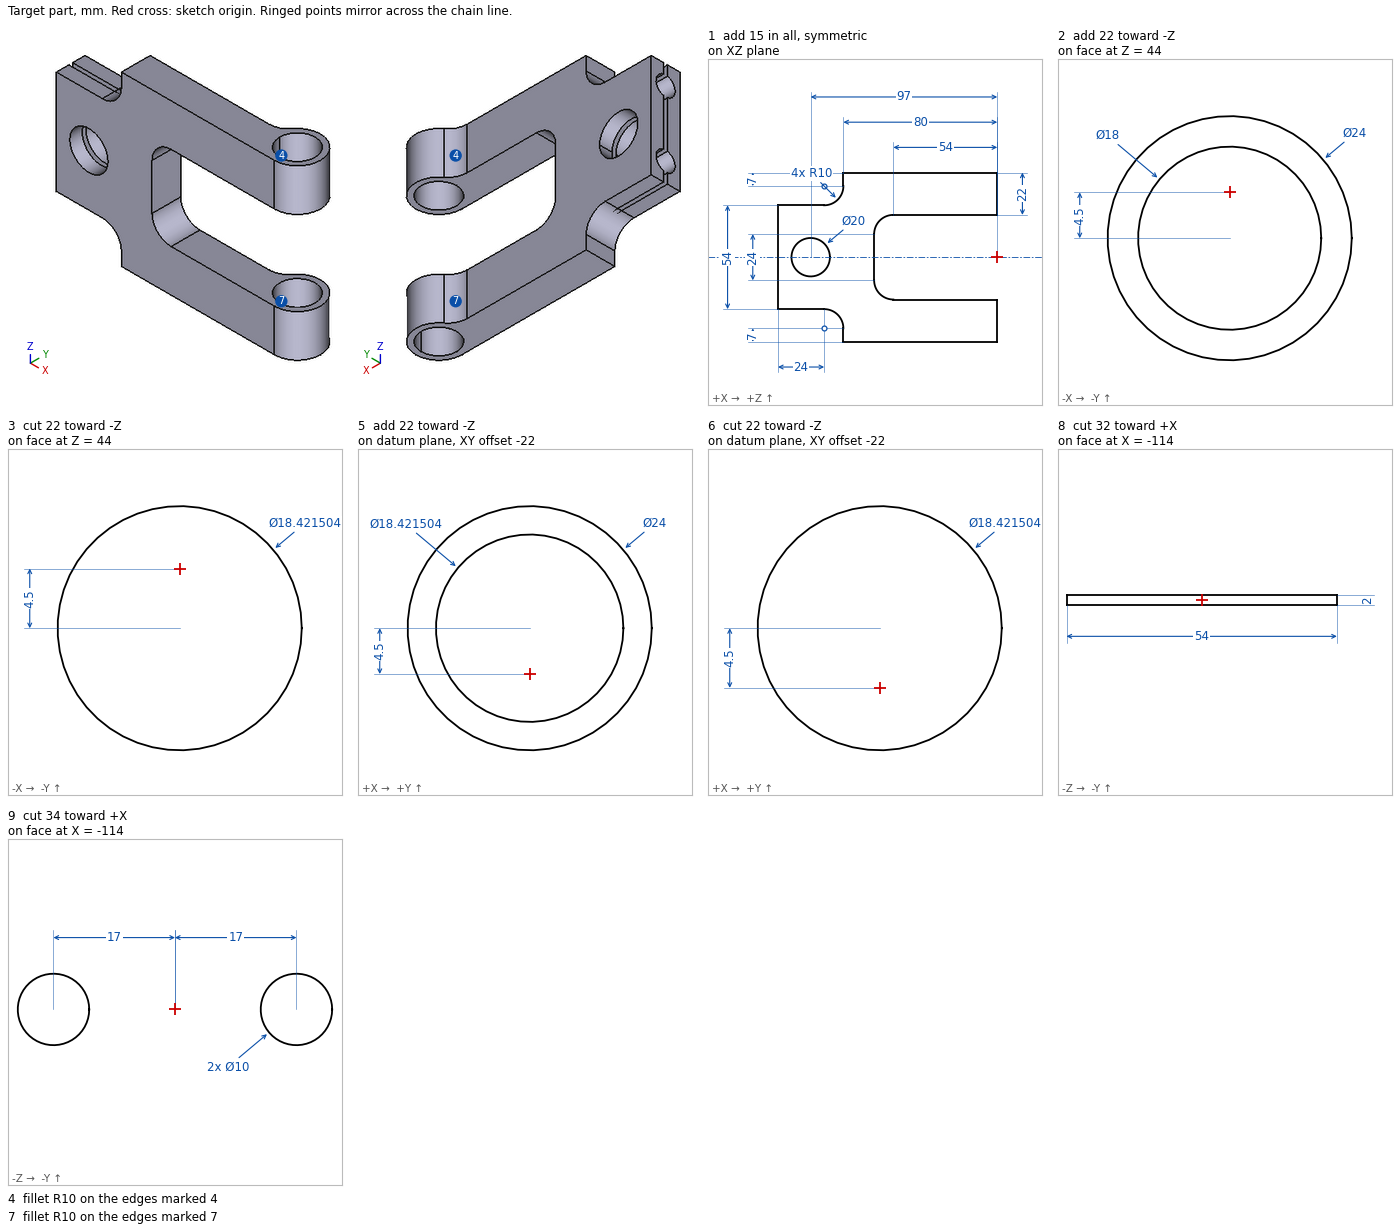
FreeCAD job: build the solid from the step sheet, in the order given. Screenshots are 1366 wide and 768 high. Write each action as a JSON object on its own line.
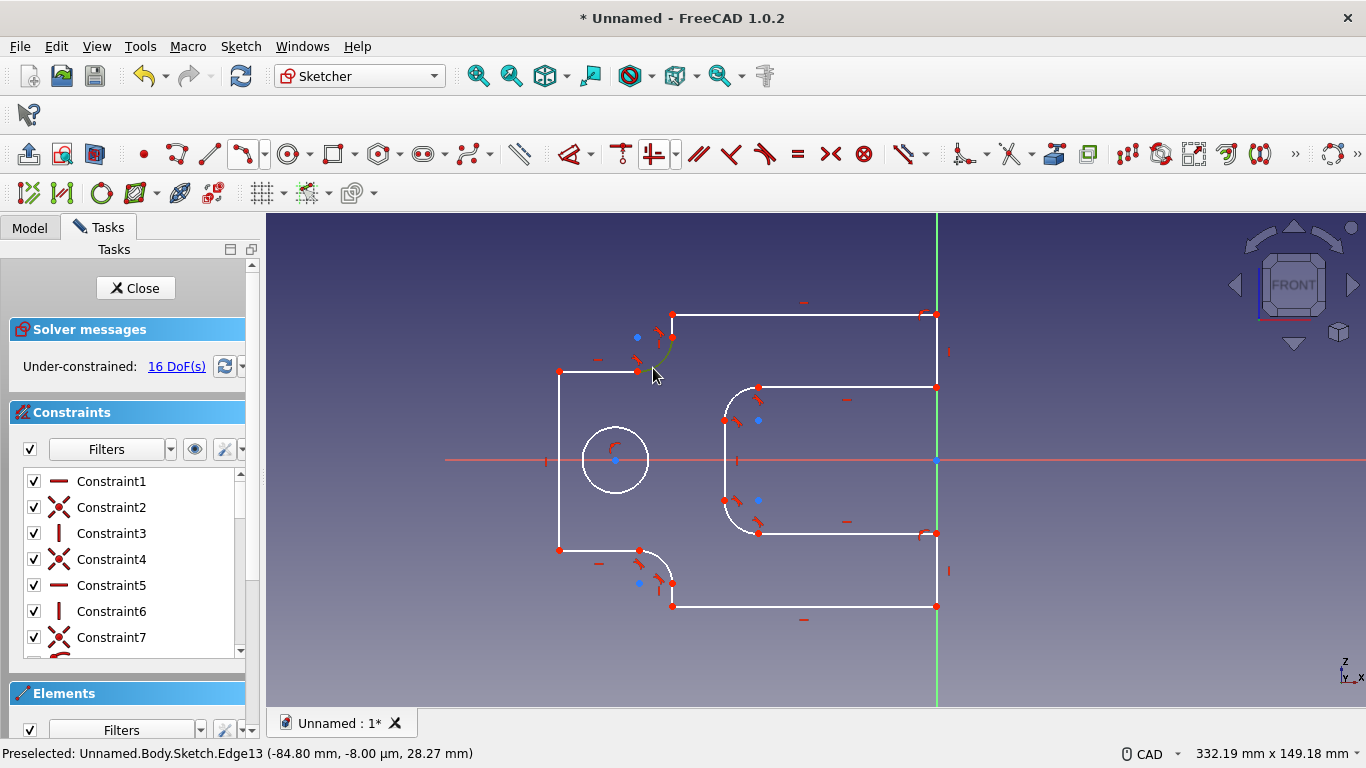
{"action": "left_click", "coordinate": [743, 391]}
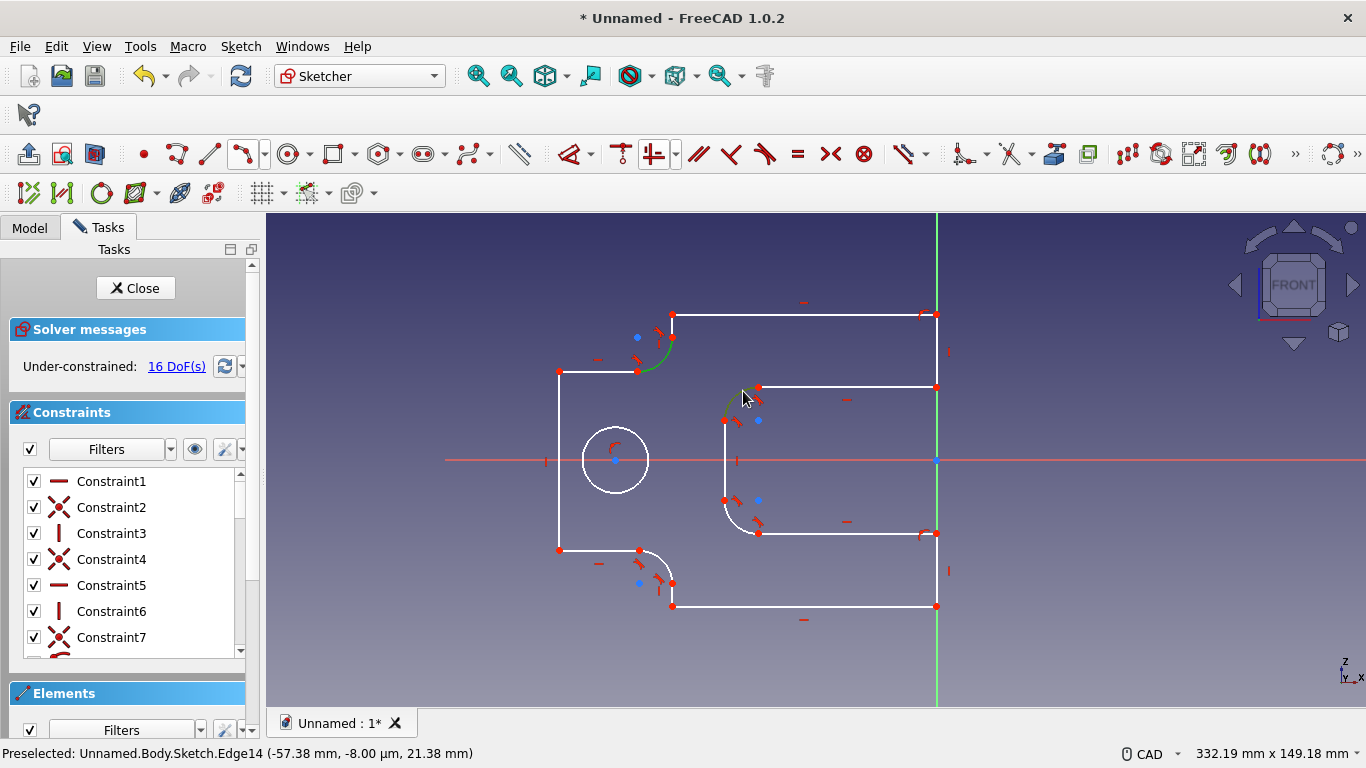
{"action": "left_click", "coordinate": [728, 516]}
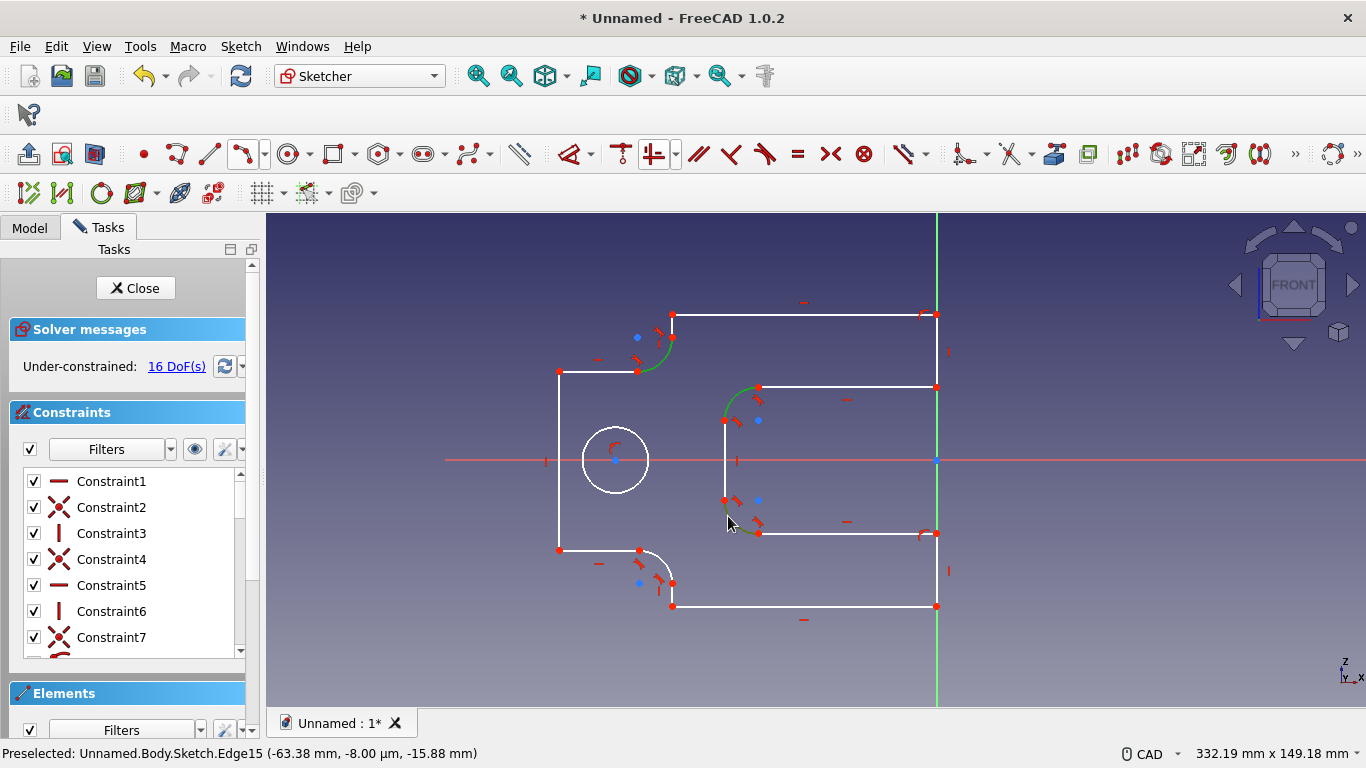
{"action": "left_click", "coordinate": [669, 569]}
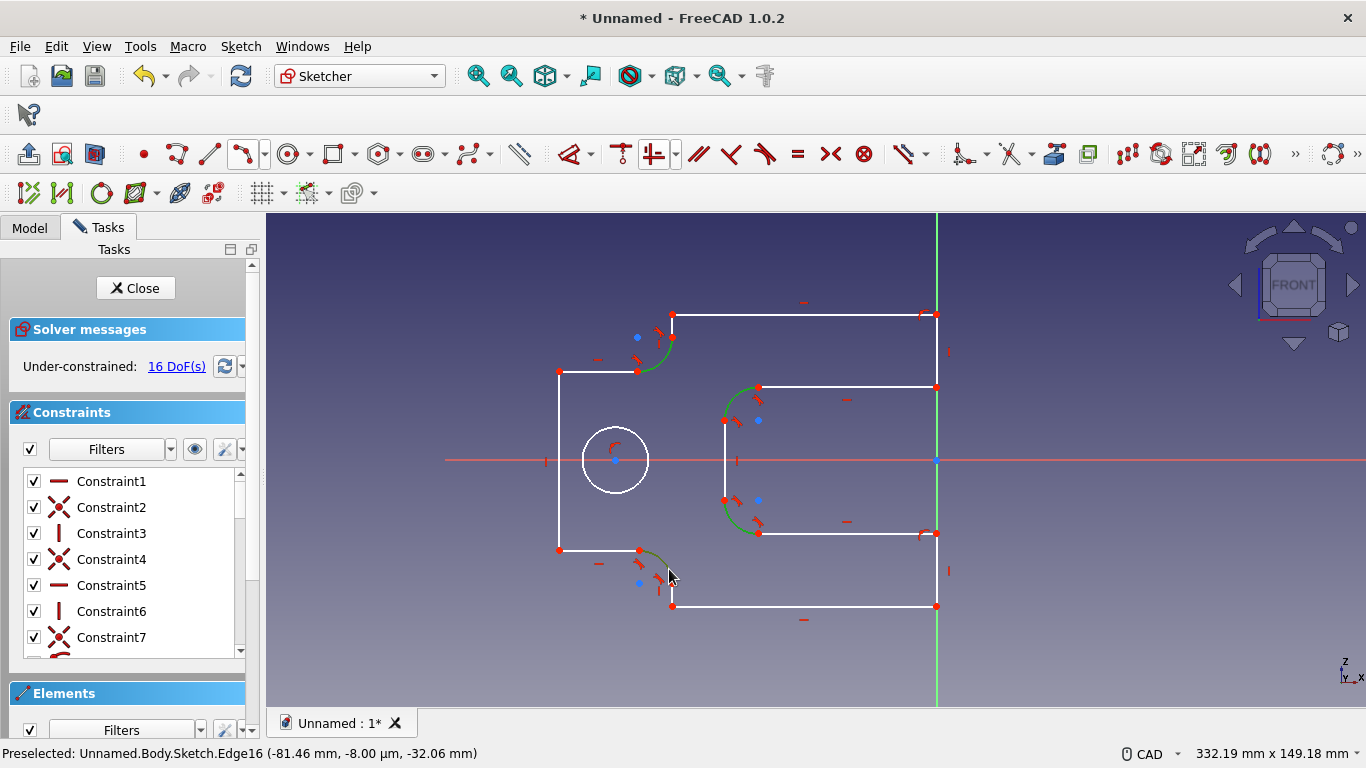
{"action": "left_click", "coordinate": [798, 154]}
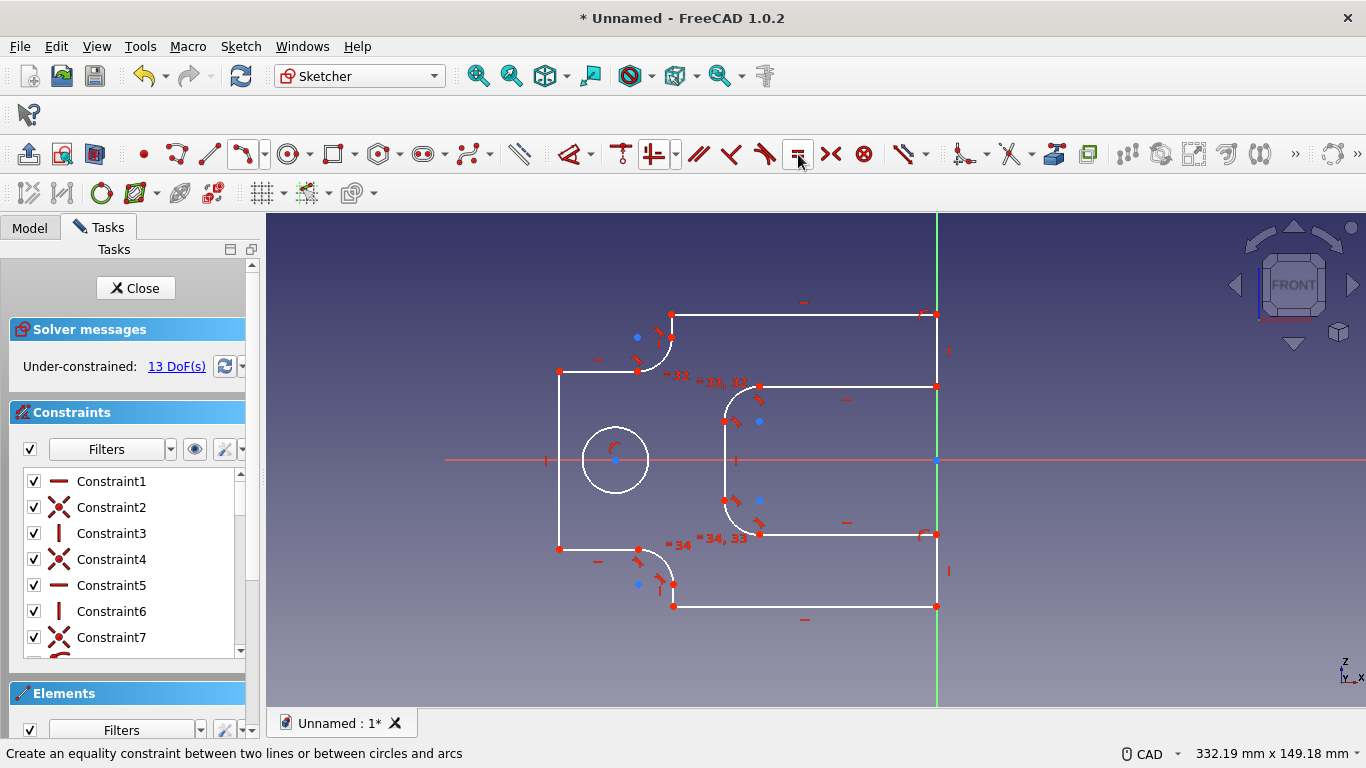
{"action": "left_click", "coordinate": [637, 337]}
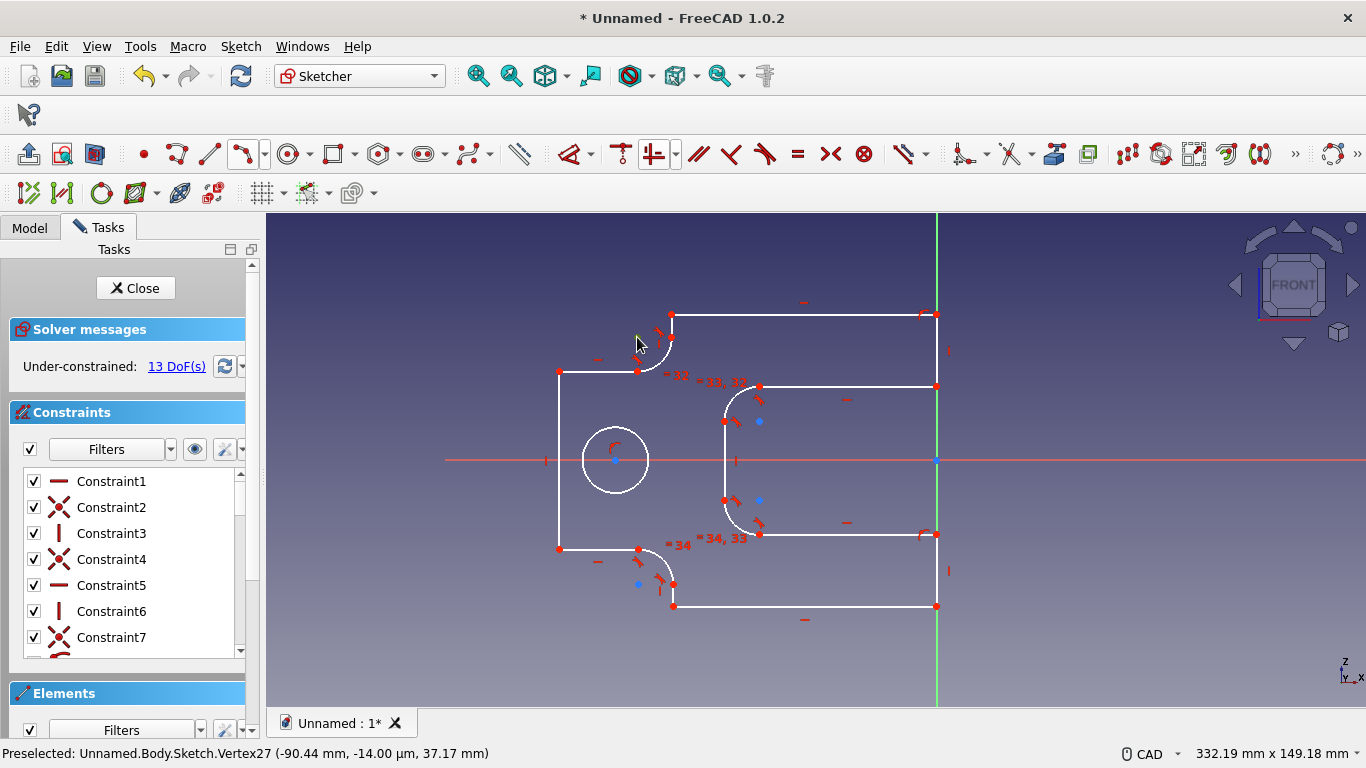
{"action": "left_click", "coordinate": [639, 584]}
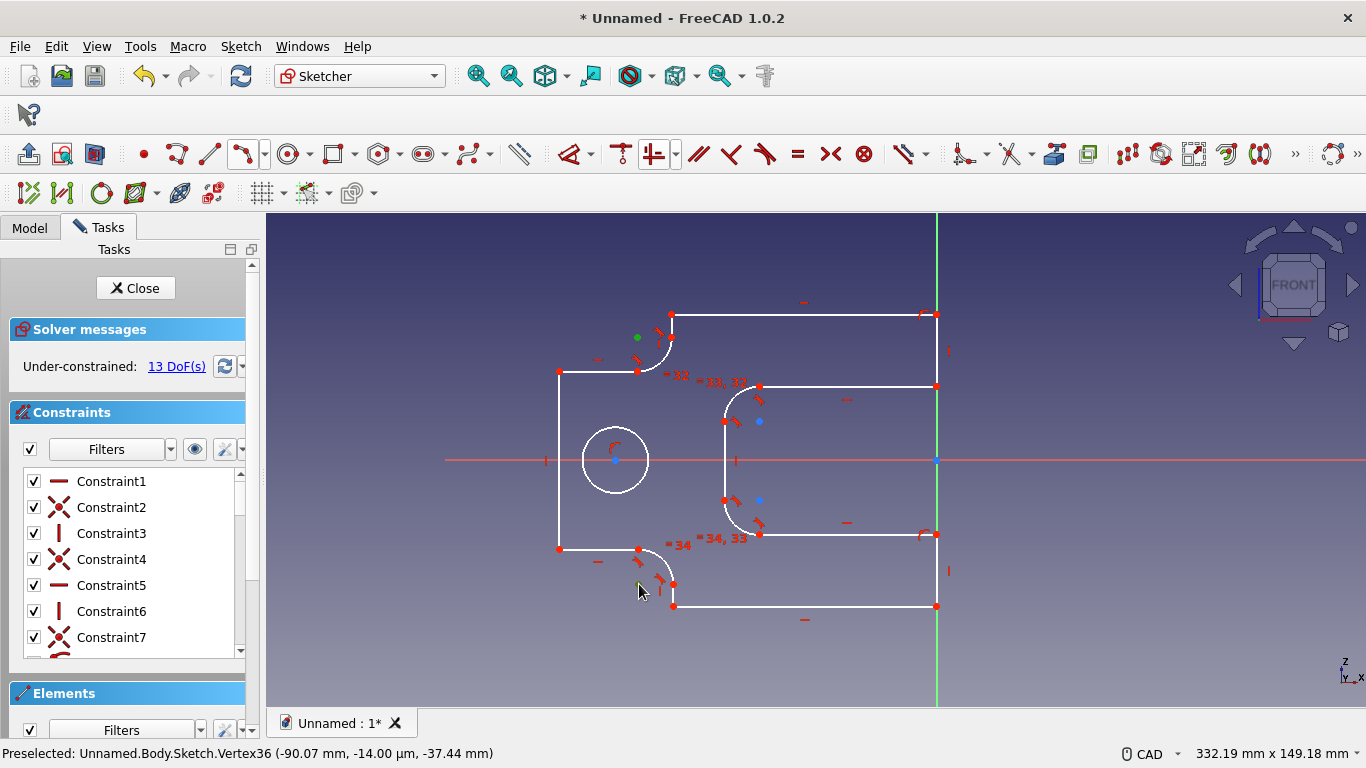
{"action": "left_click", "coordinate": [488, 460]}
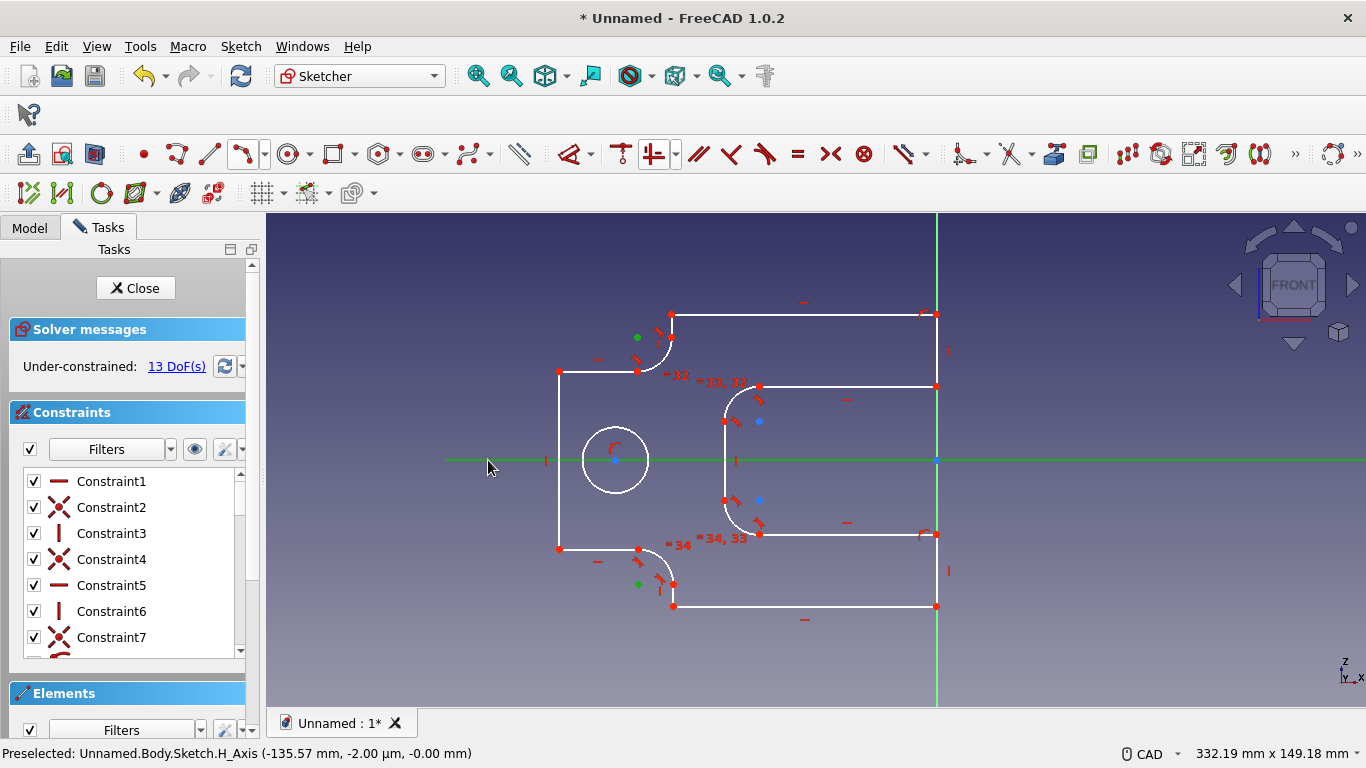
{"action": "left_click", "coordinate": [831, 154]}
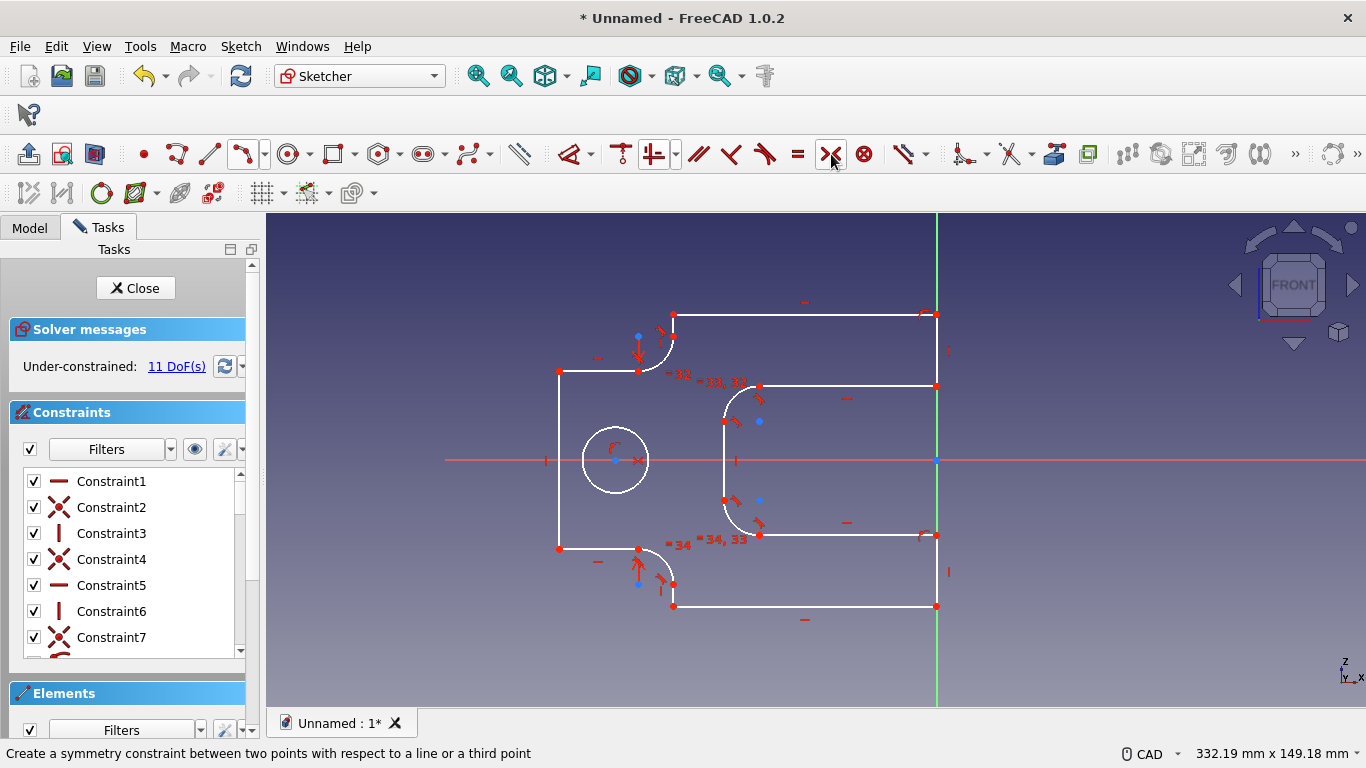
{"action": "left_click", "coordinate": [568, 154]}